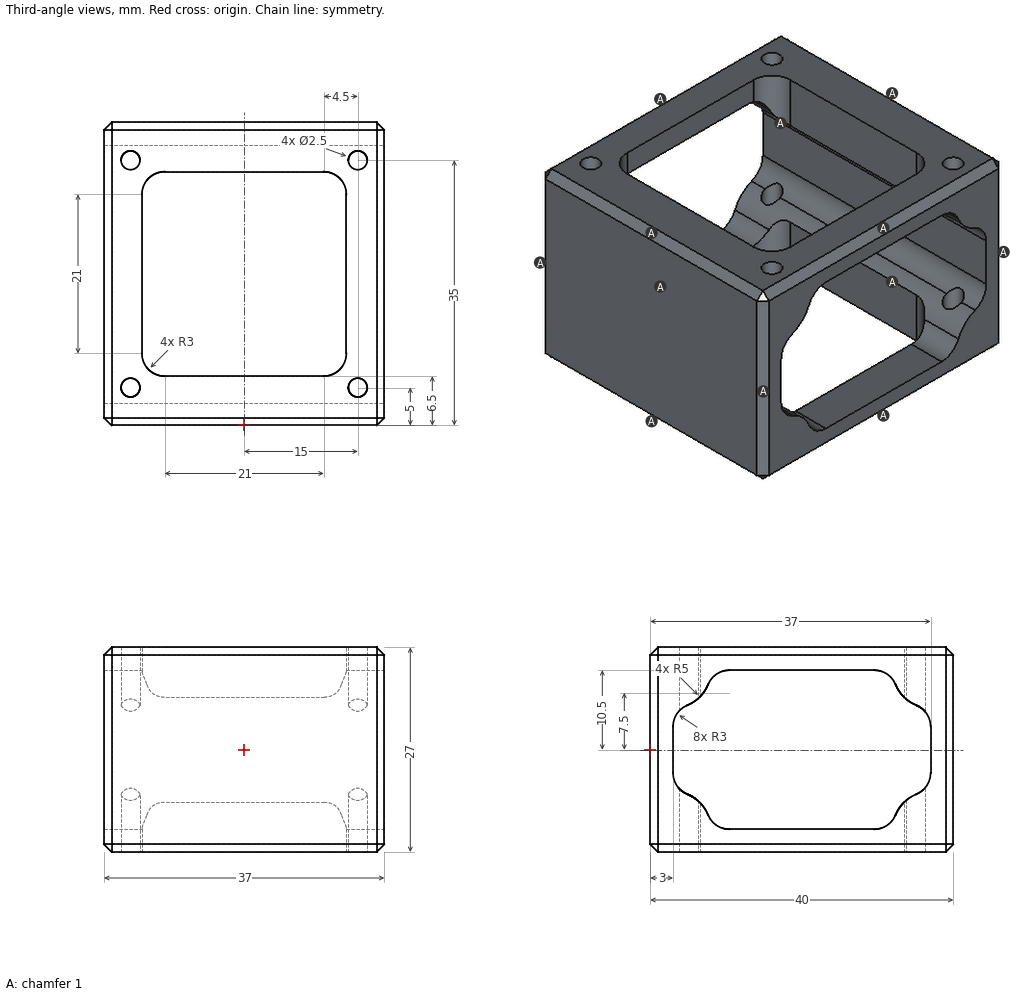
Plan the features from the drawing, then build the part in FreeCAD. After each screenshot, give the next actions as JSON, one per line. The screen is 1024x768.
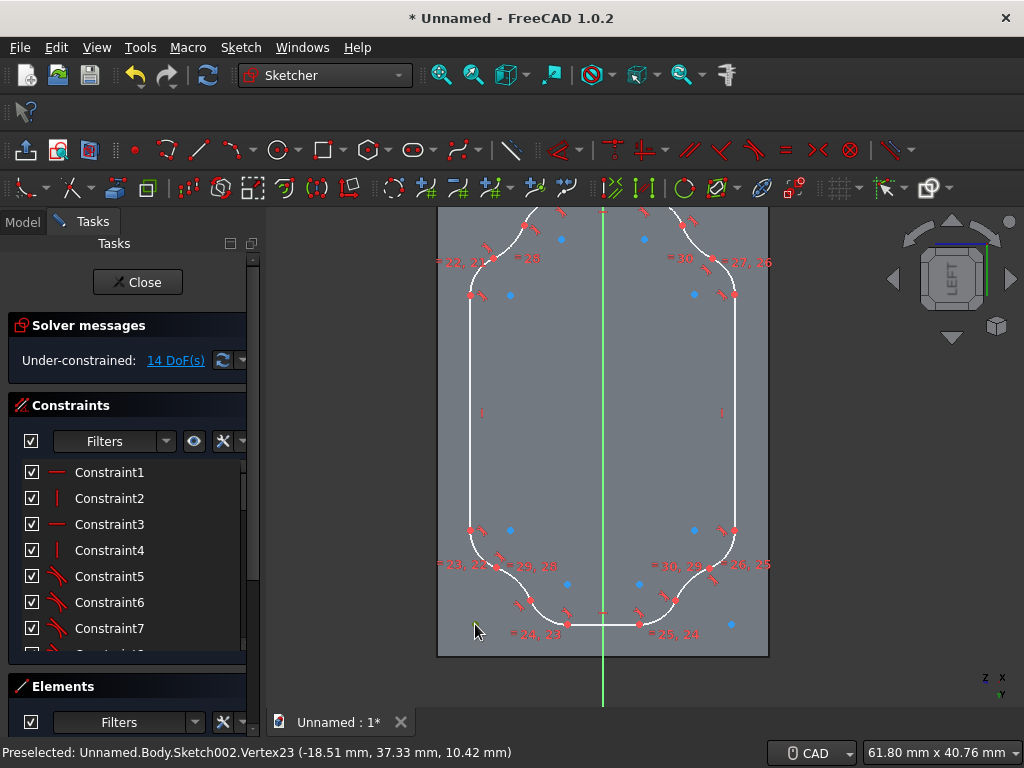
{"action": "left_click", "coordinate": [731, 624]}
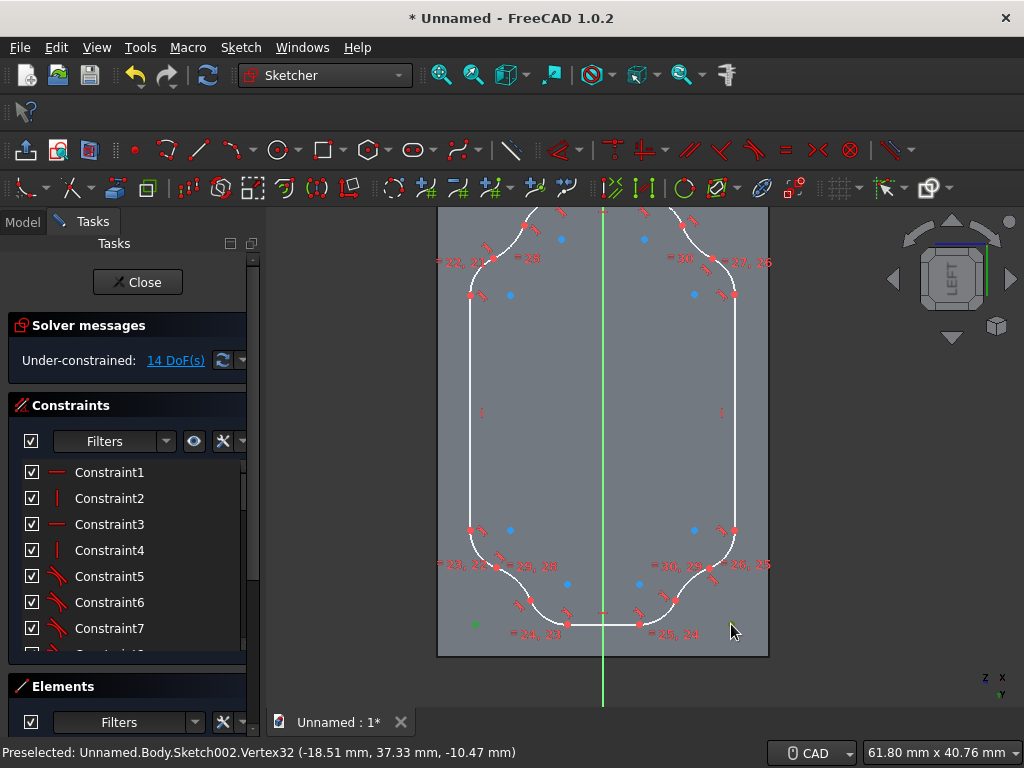
{"action": "left_click", "coordinate": [603, 584]}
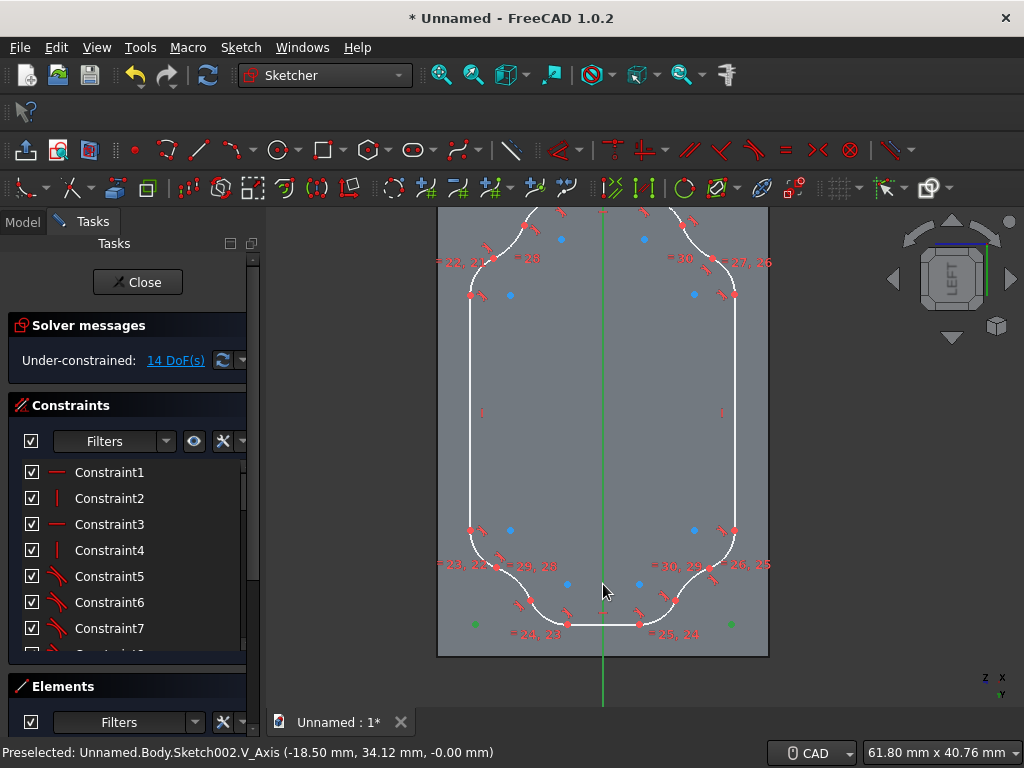
{"action": "key", "text": "s"}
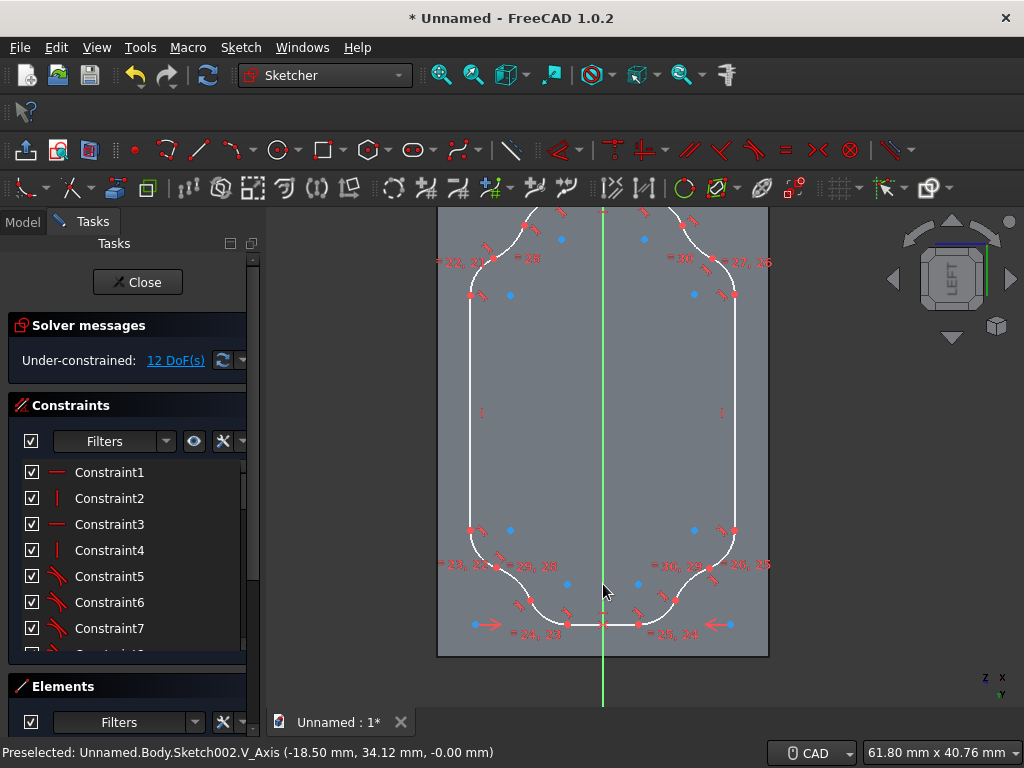
{"action": "left_click", "coordinate": [510, 295]}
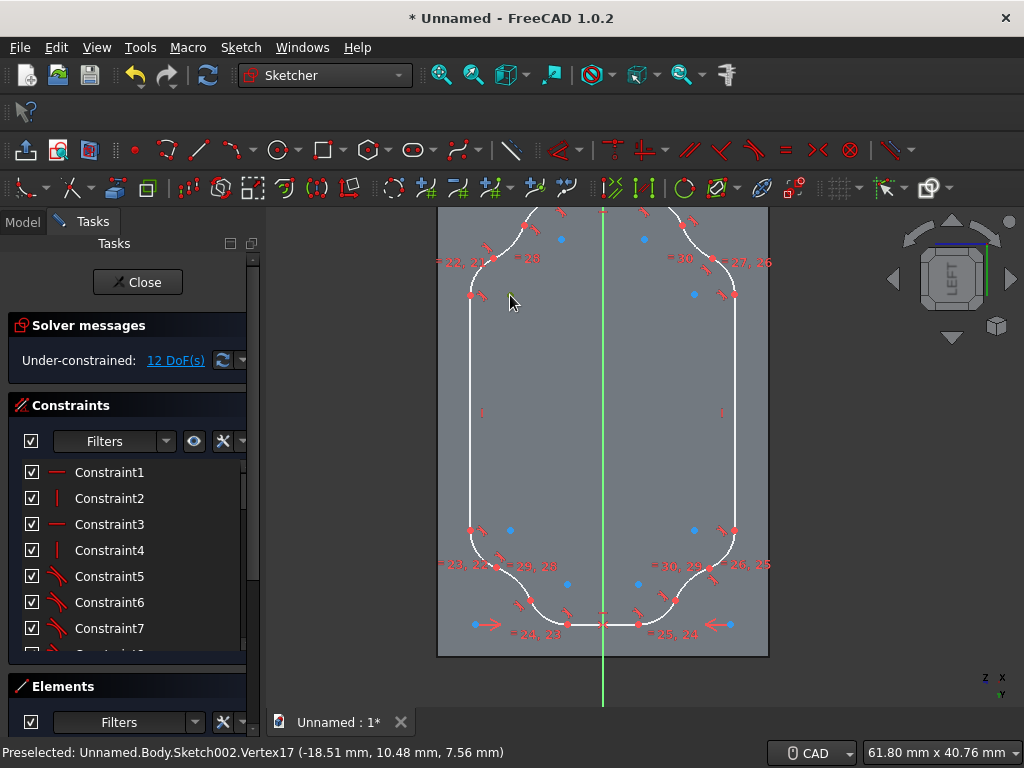
{"action": "left_click", "coordinate": [695, 295]}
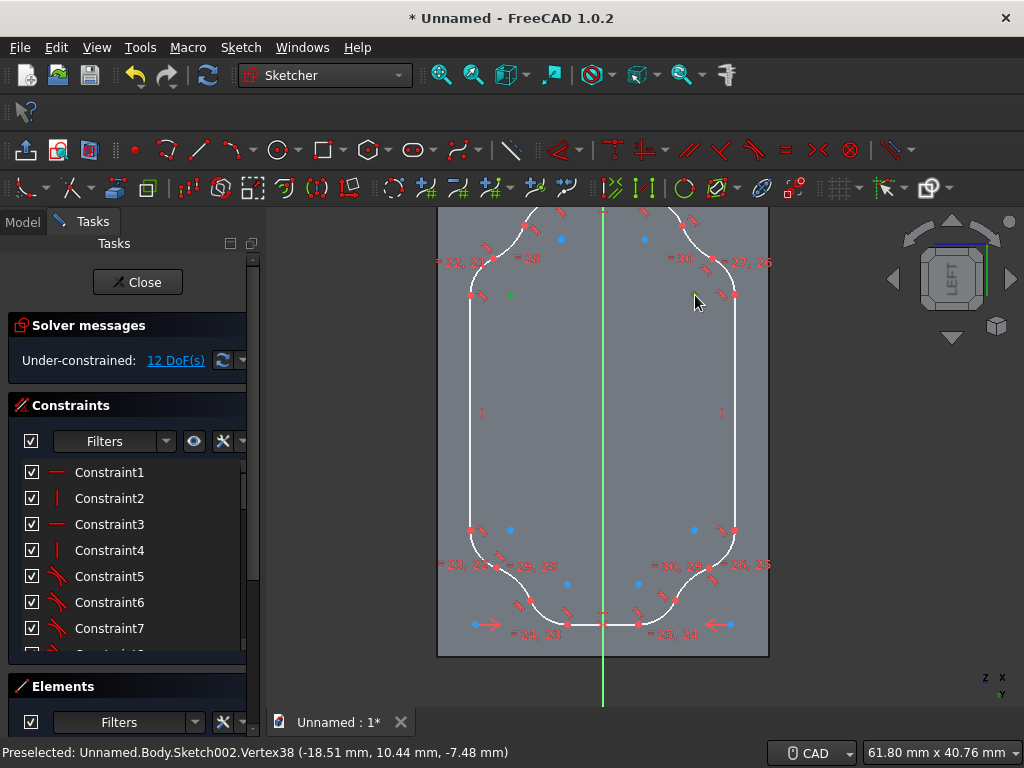
{"action": "left_click", "coordinate": [603, 584]}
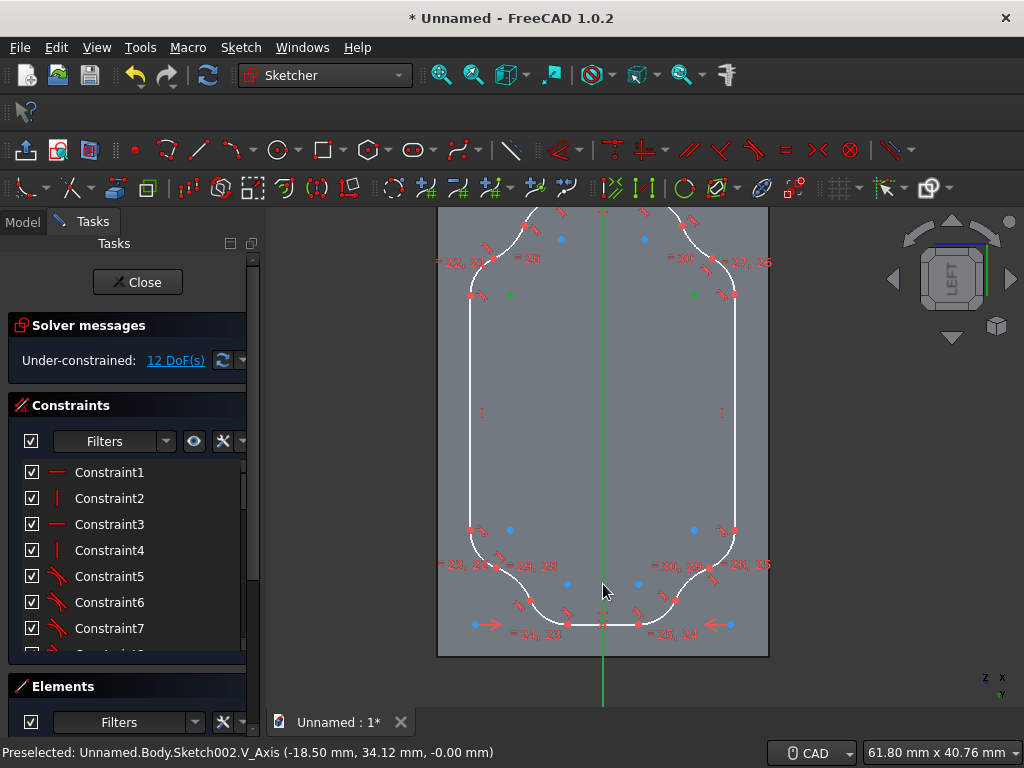
{"action": "key", "text": "s"}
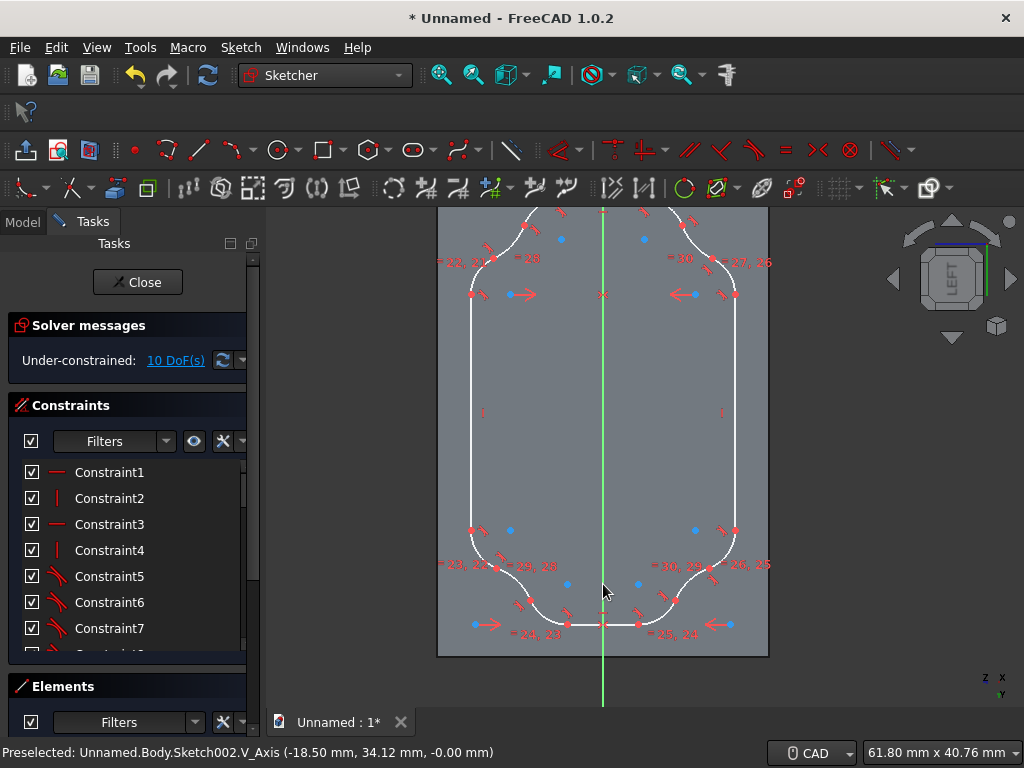
{"action": "key", "text": "d"}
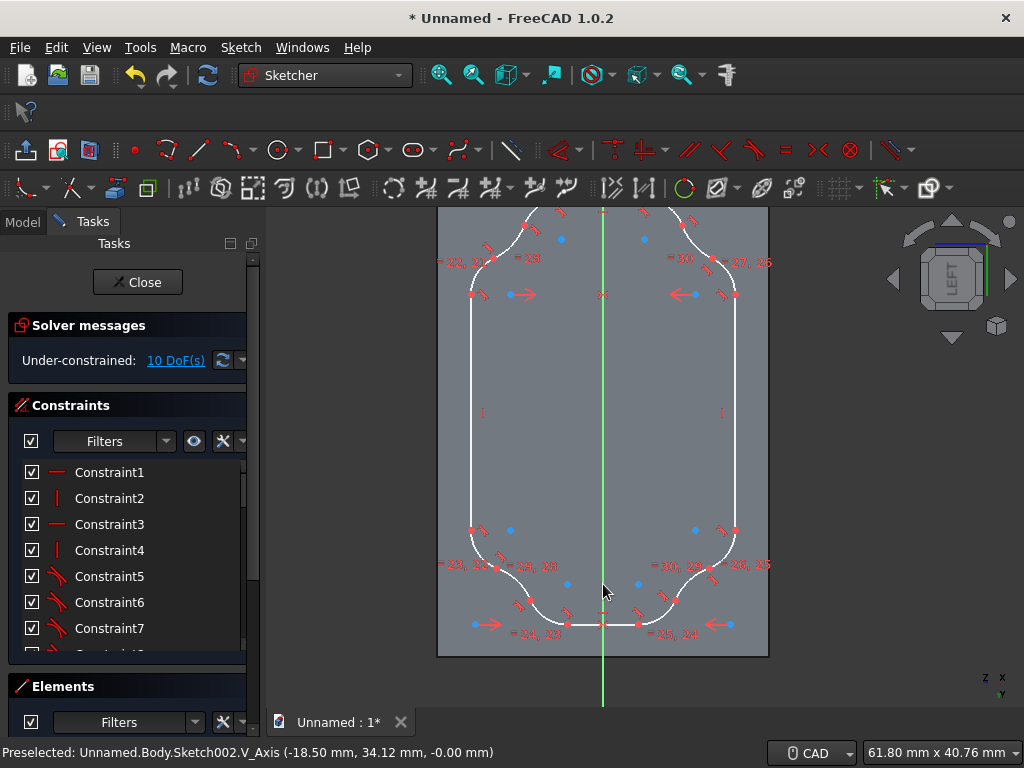
{"action": "scroll", "coordinate": [523, 586], "scroll_direction": "down", "scroll_amount": 2}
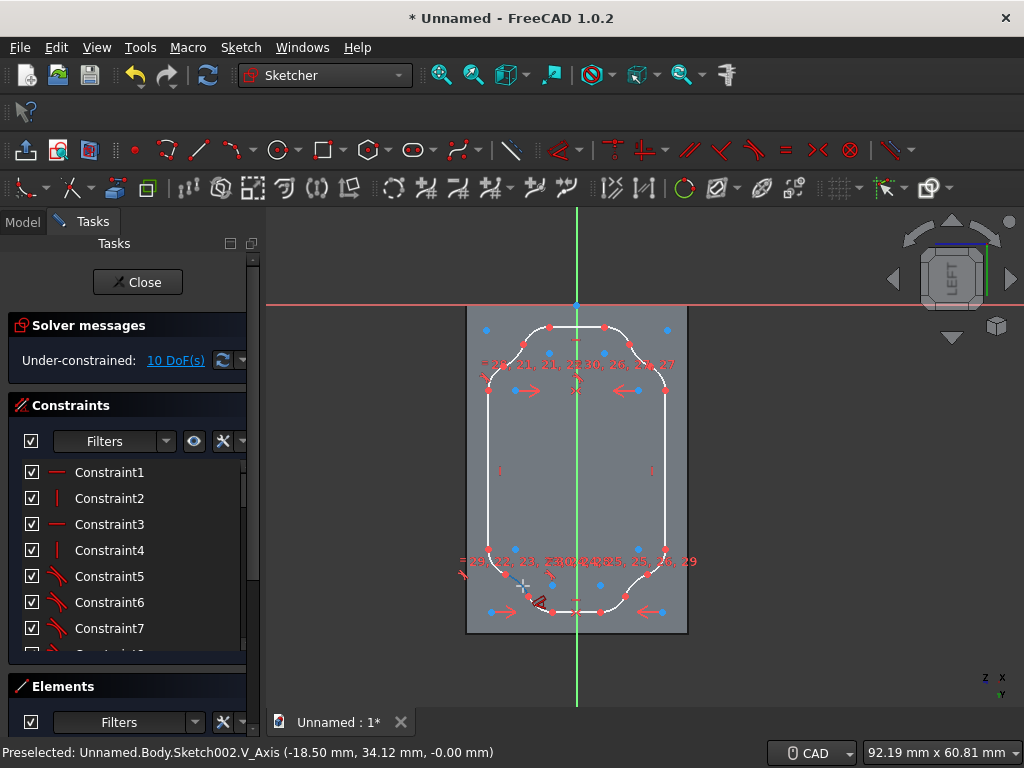
{"action": "scroll", "coordinate": [540, 329], "scroll_direction": "up", "scroll_amount": 3}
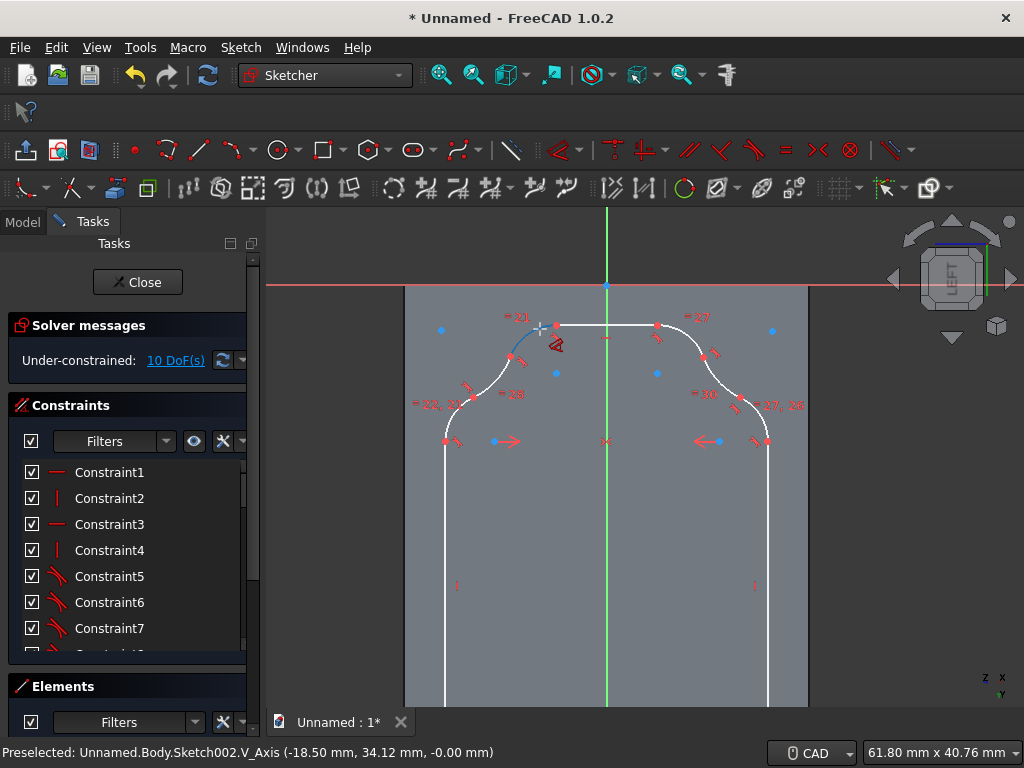
{"action": "left_click", "coordinate": [539, 328]}
{"action": "left_click", "coordinate": [495, 321]}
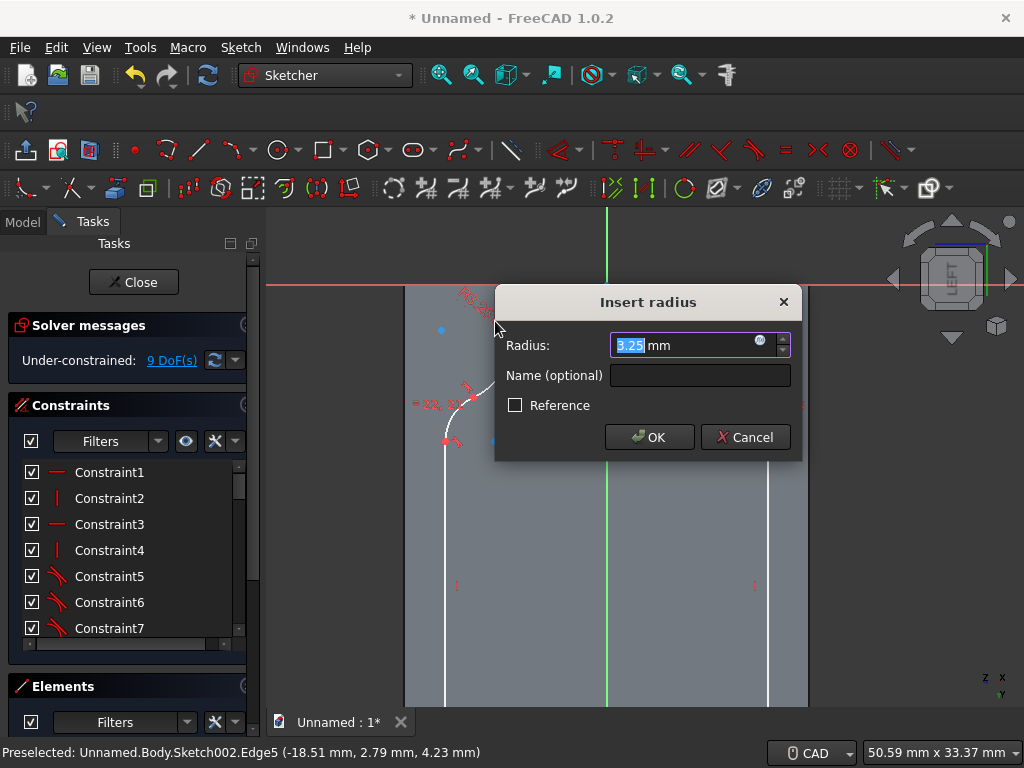
{"action": "type", "text": "3"}
{"action": "key", "text": "Return"}